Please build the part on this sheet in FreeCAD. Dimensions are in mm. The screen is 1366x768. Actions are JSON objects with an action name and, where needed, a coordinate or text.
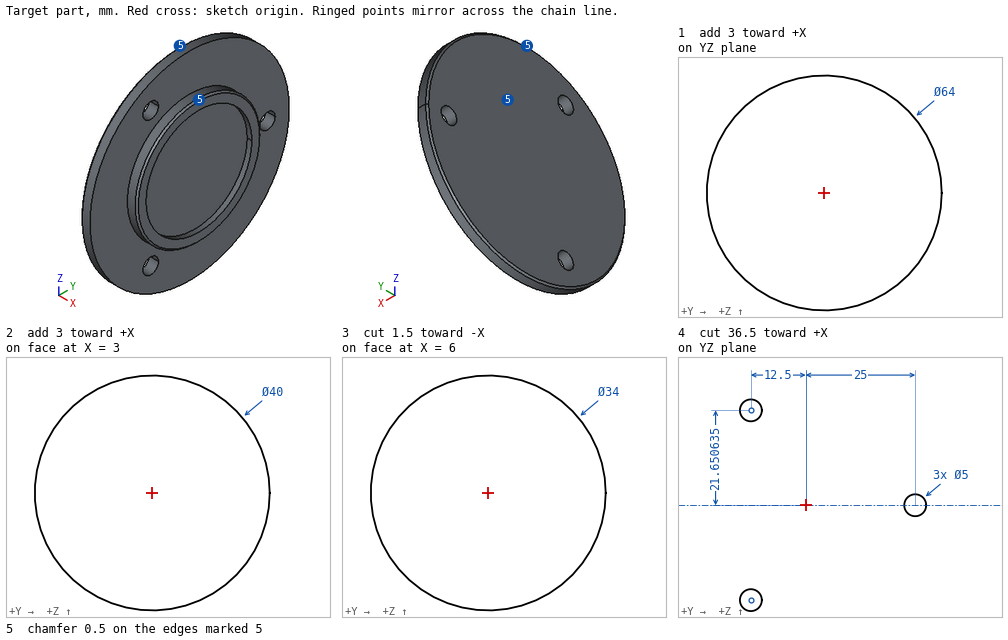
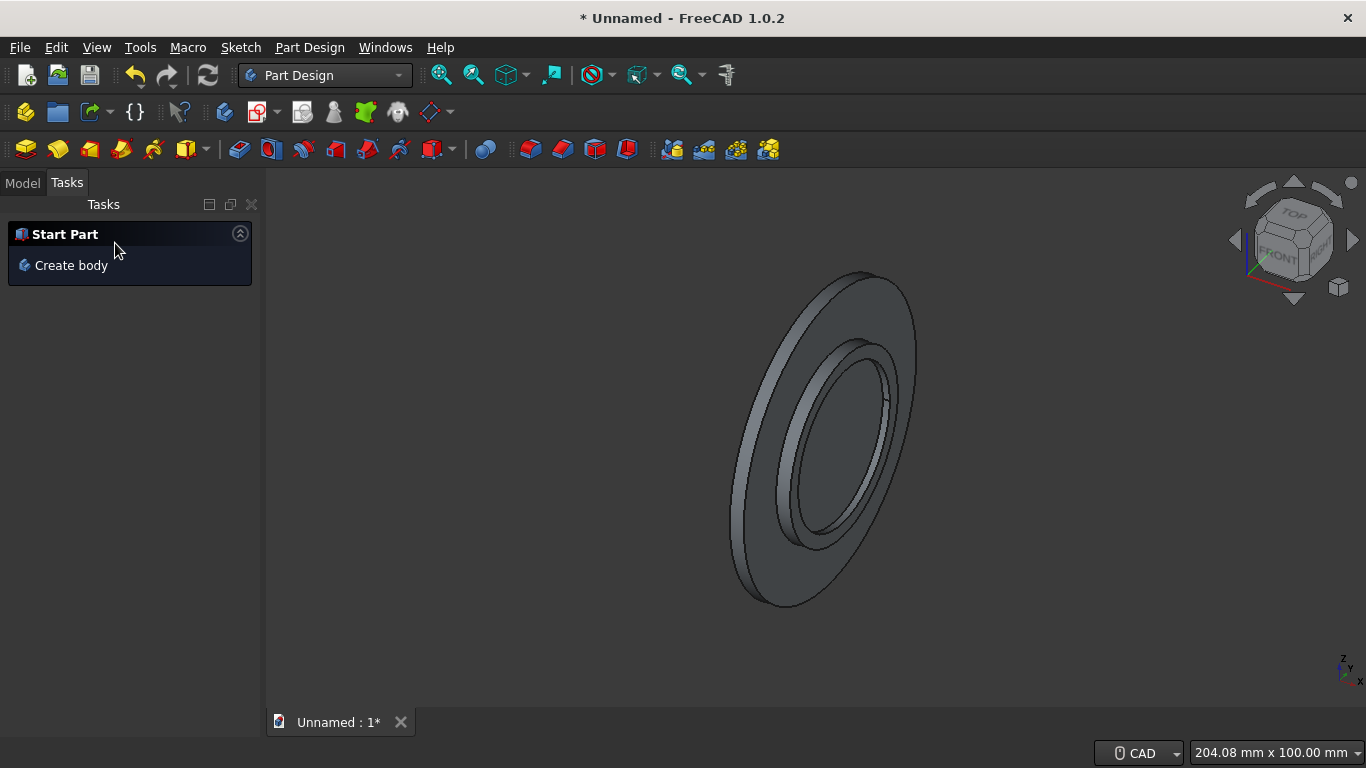
{"action": "left_click", "coordinate": [258, 112]}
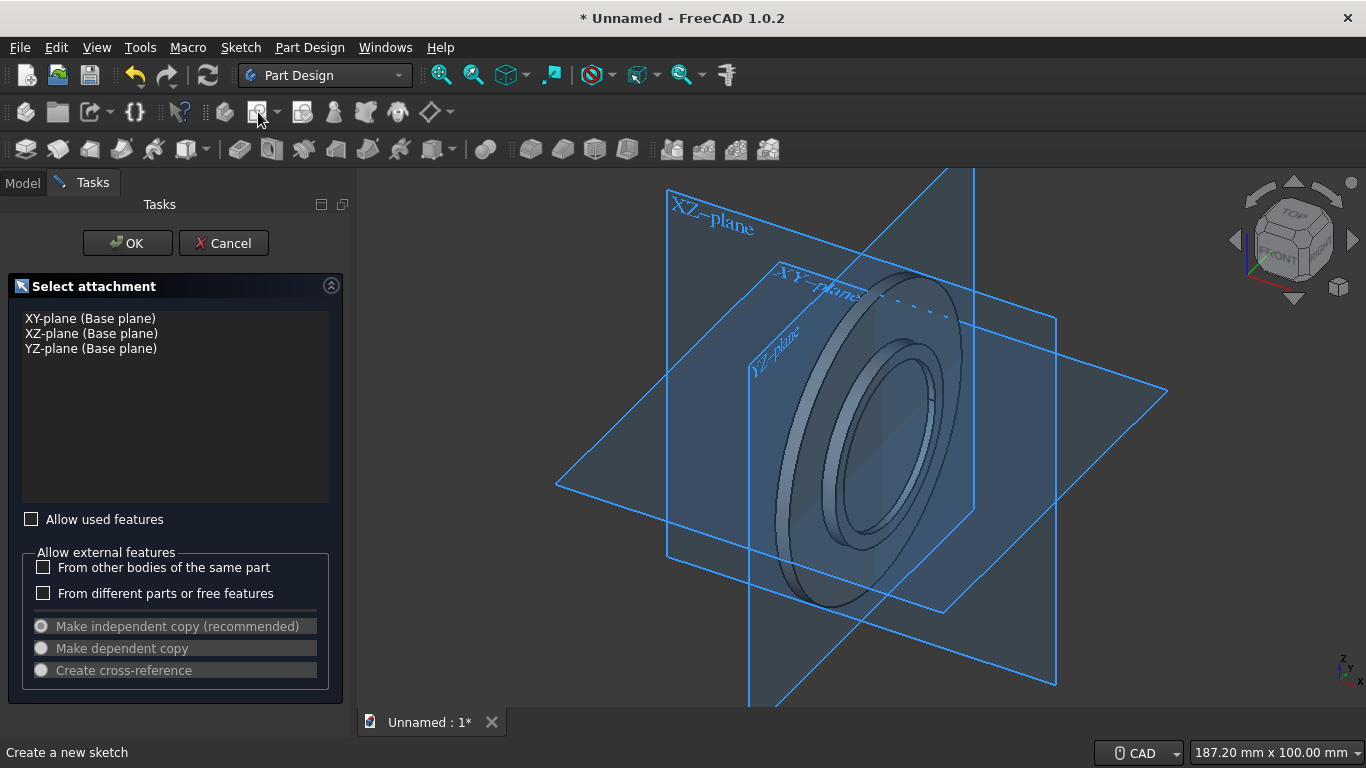
{"action": "left_click", "coordinate": [82, 348]}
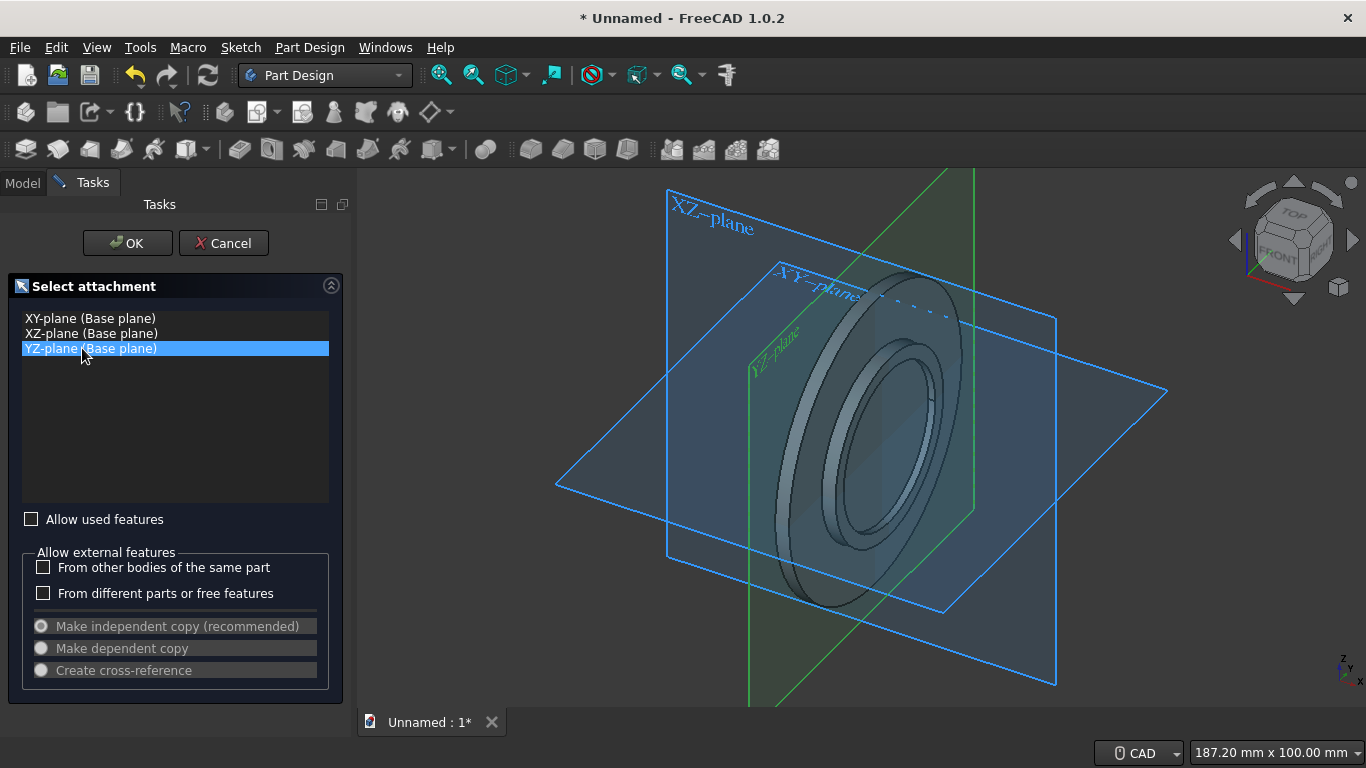
{"action": "left_click", "coordinate": [128, 243]}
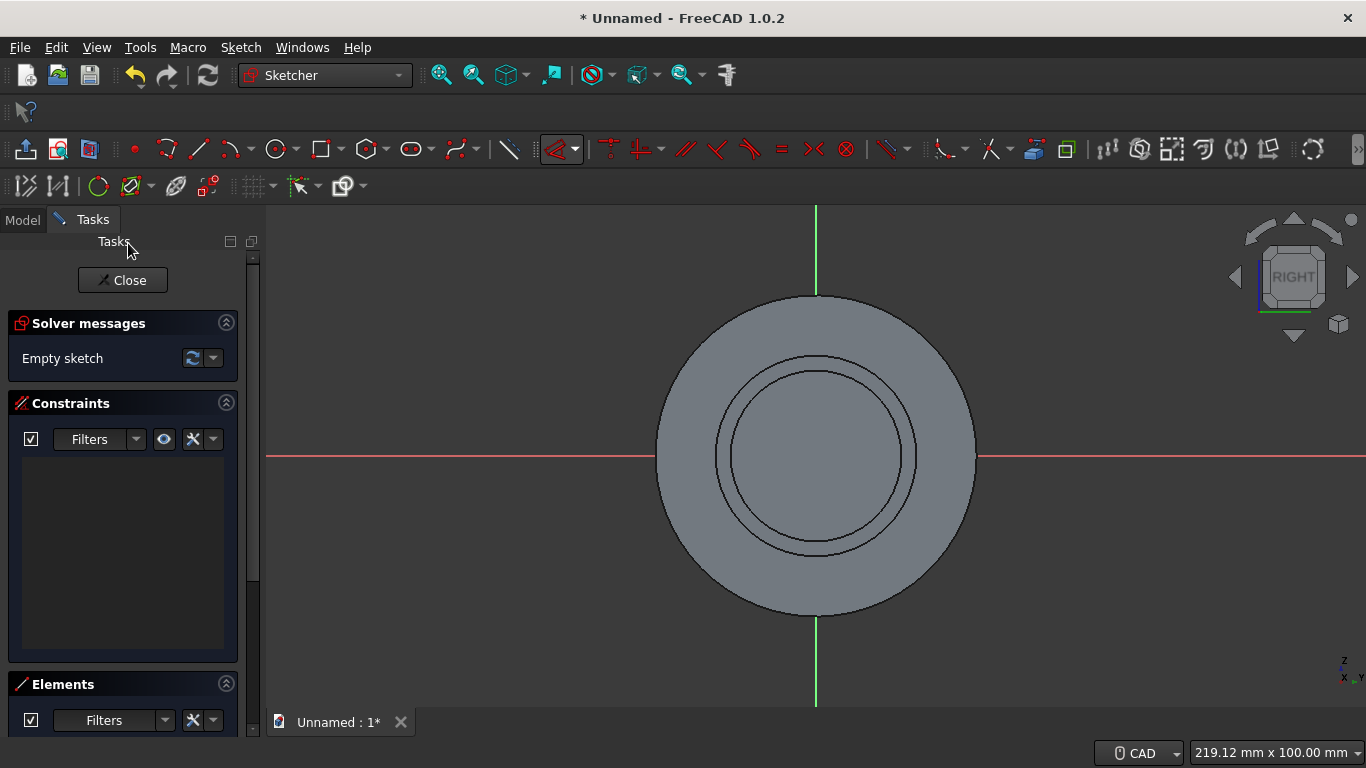
{"action": "left_click", "coordinate": [90, 150]}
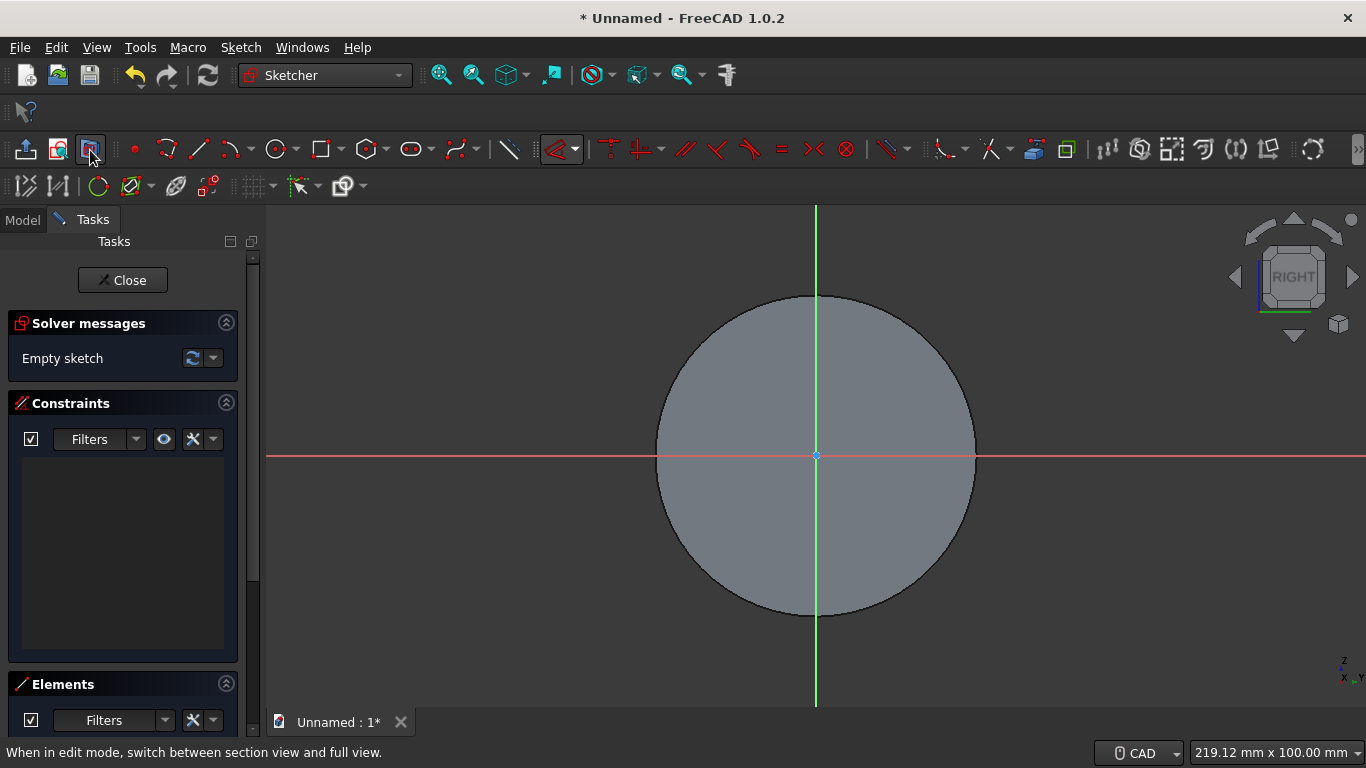
{"action": "left_click", "coordinate": [276, 150]}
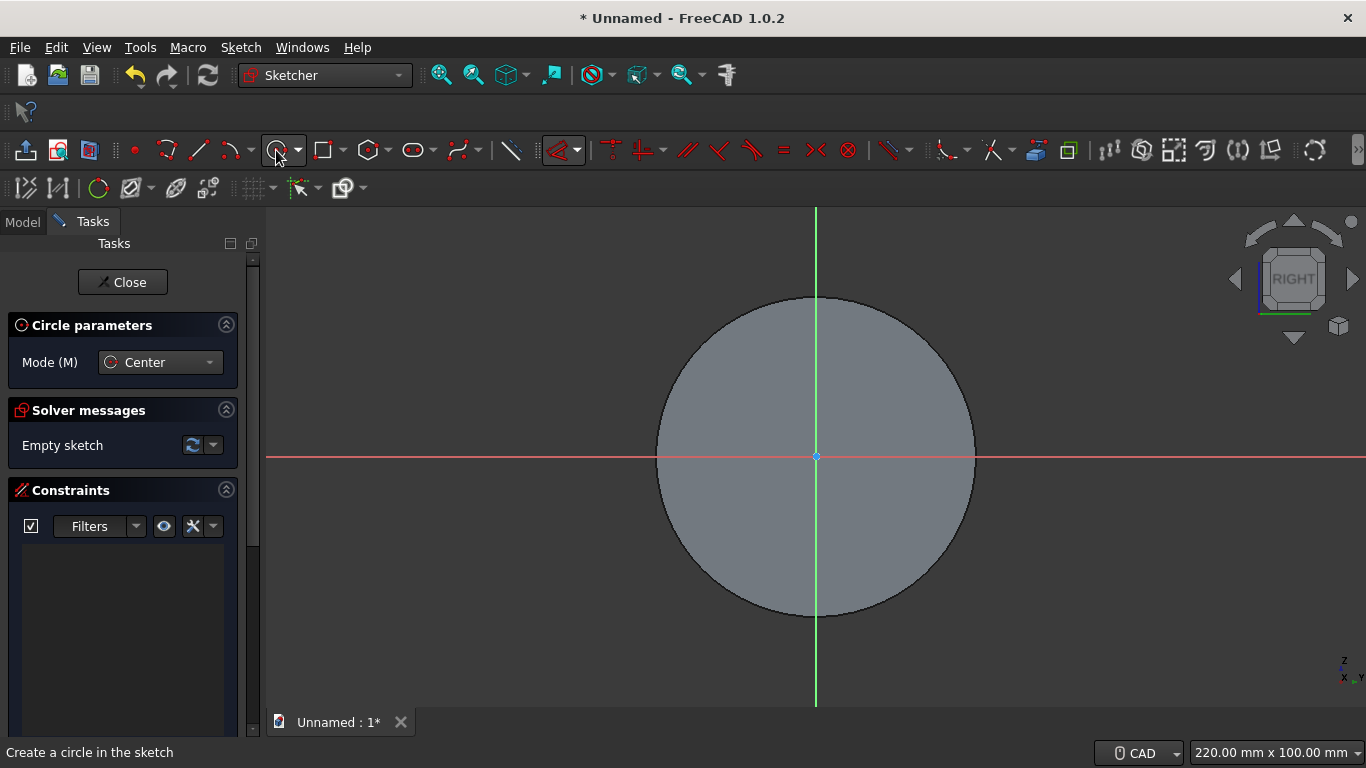
{"action": "scroll", "coordinate": [941, 457], "scroll_direction": "up", "scroll_amount": 3}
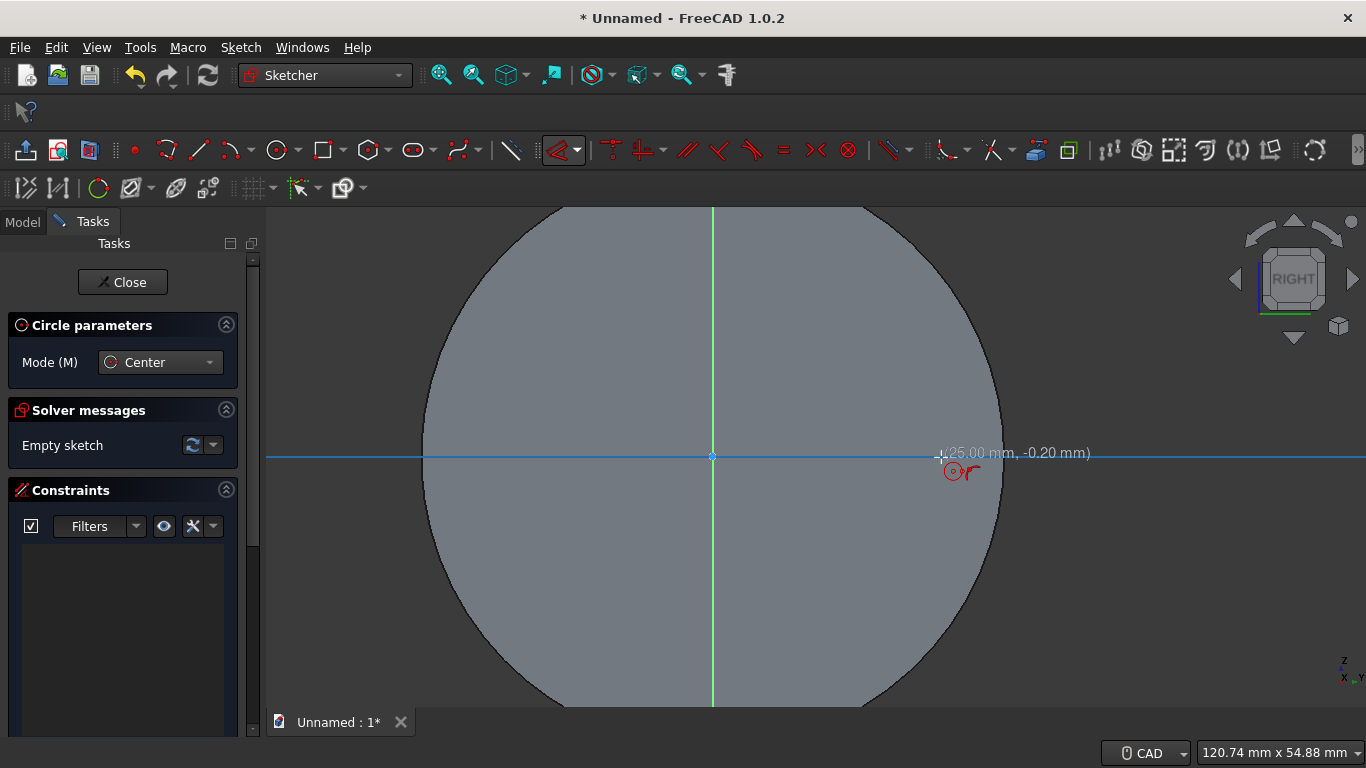
{"action": "left_click", "coordinate": [940, 457]}
{"action": "left_click", "coordinate": [957, 440]}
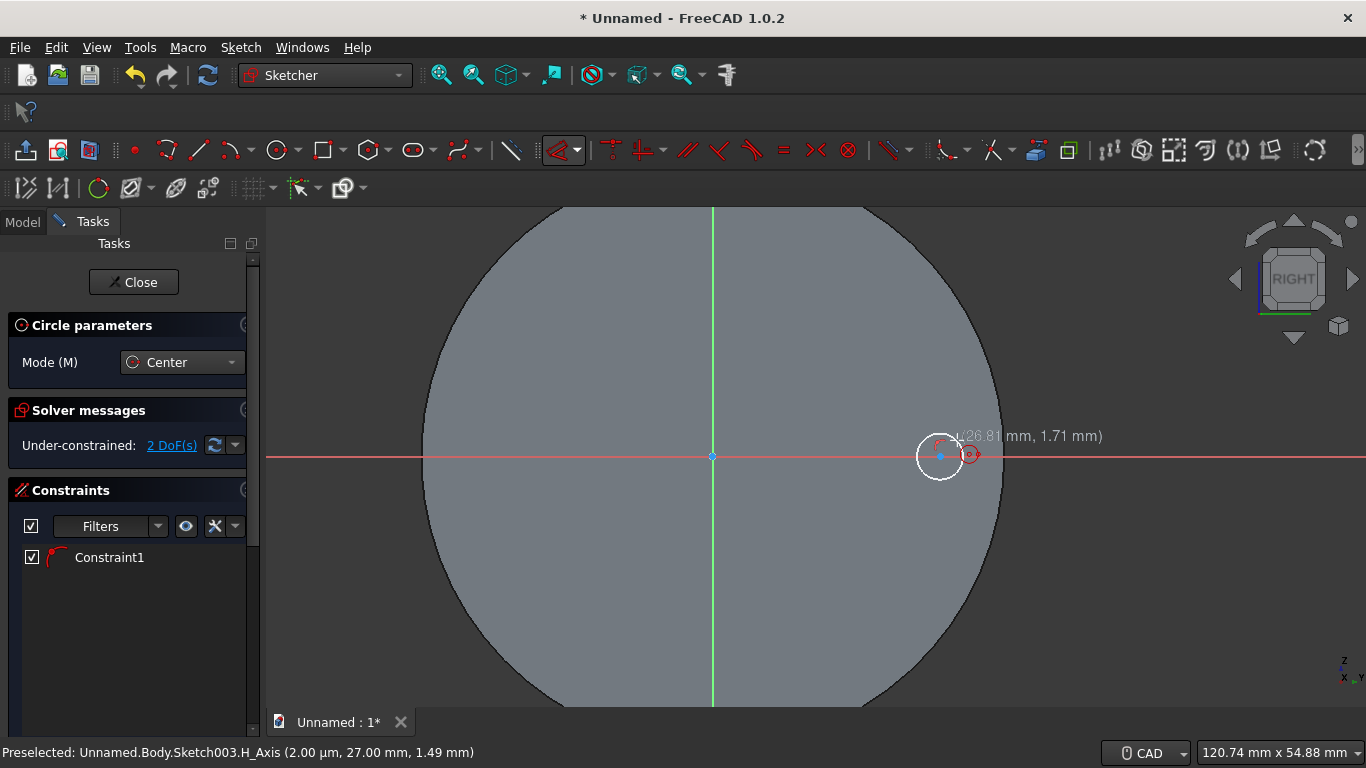
{"action": "left_click", "coordinate": [599, 259]}
{"action": "left_click", "coordinate": [615, 243]}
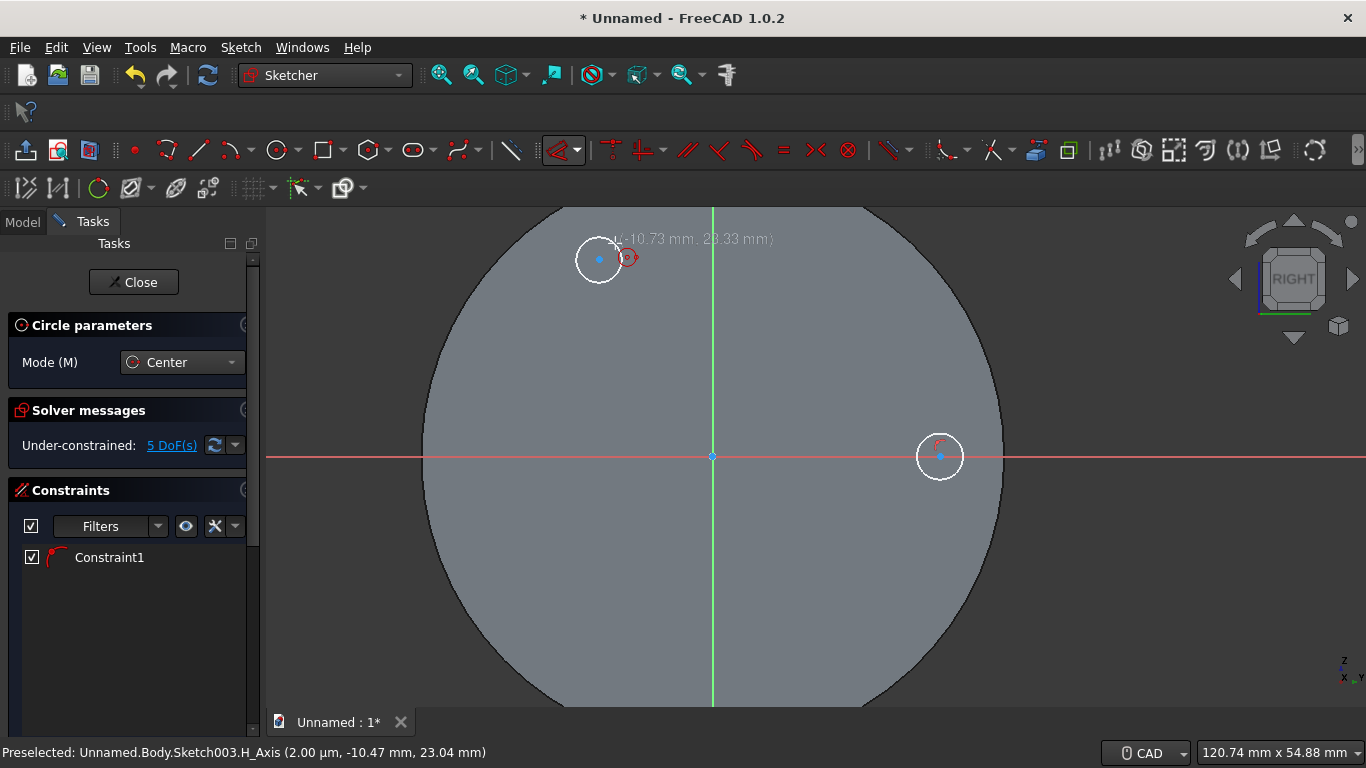
{"action": "left_click", "coordinate": [599, 654]}
{"action": "left_click", "coordinate": [615, 638]}
{"action": "key", "text": "Escape"}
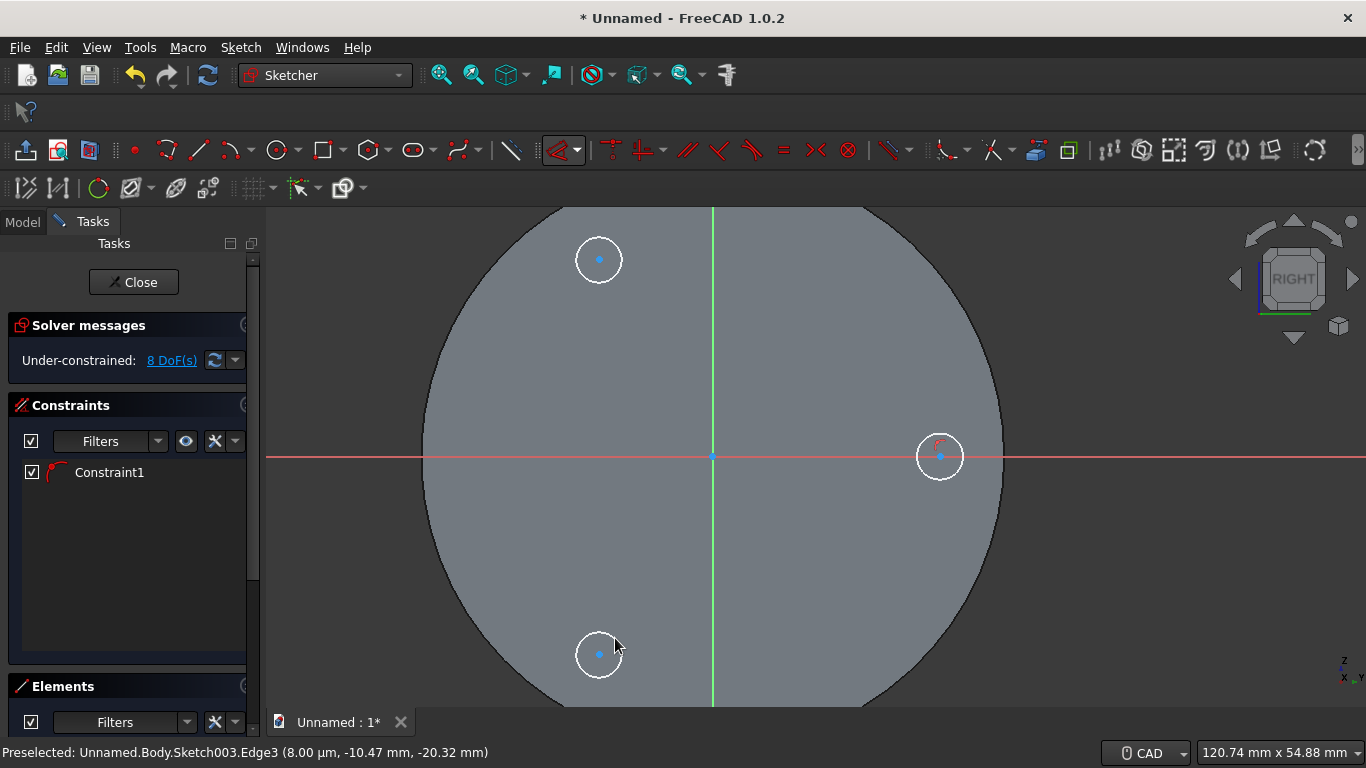
{"action": "left_click", "coordinate": [956, 440]}